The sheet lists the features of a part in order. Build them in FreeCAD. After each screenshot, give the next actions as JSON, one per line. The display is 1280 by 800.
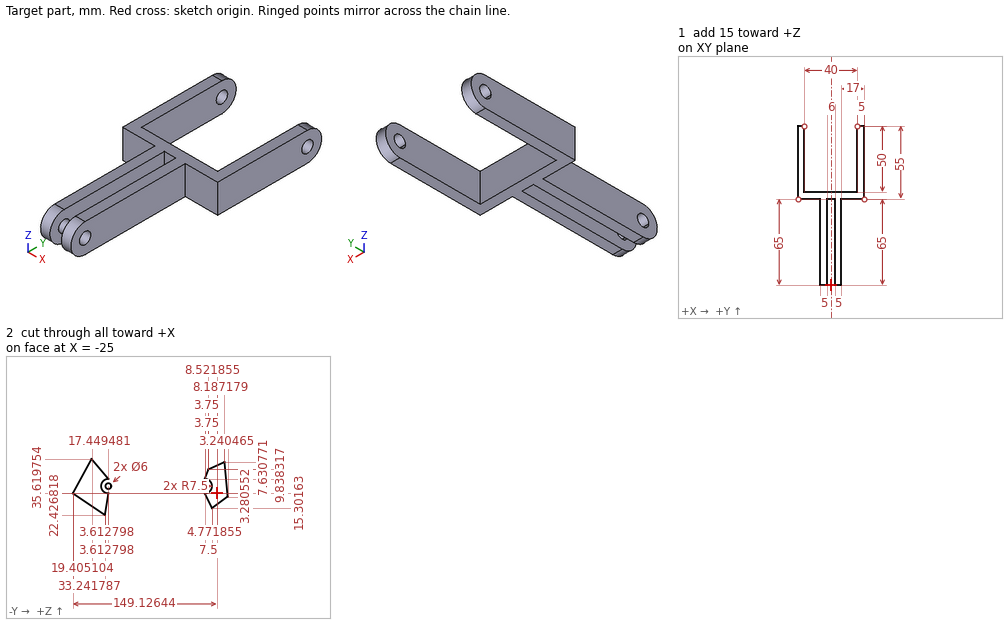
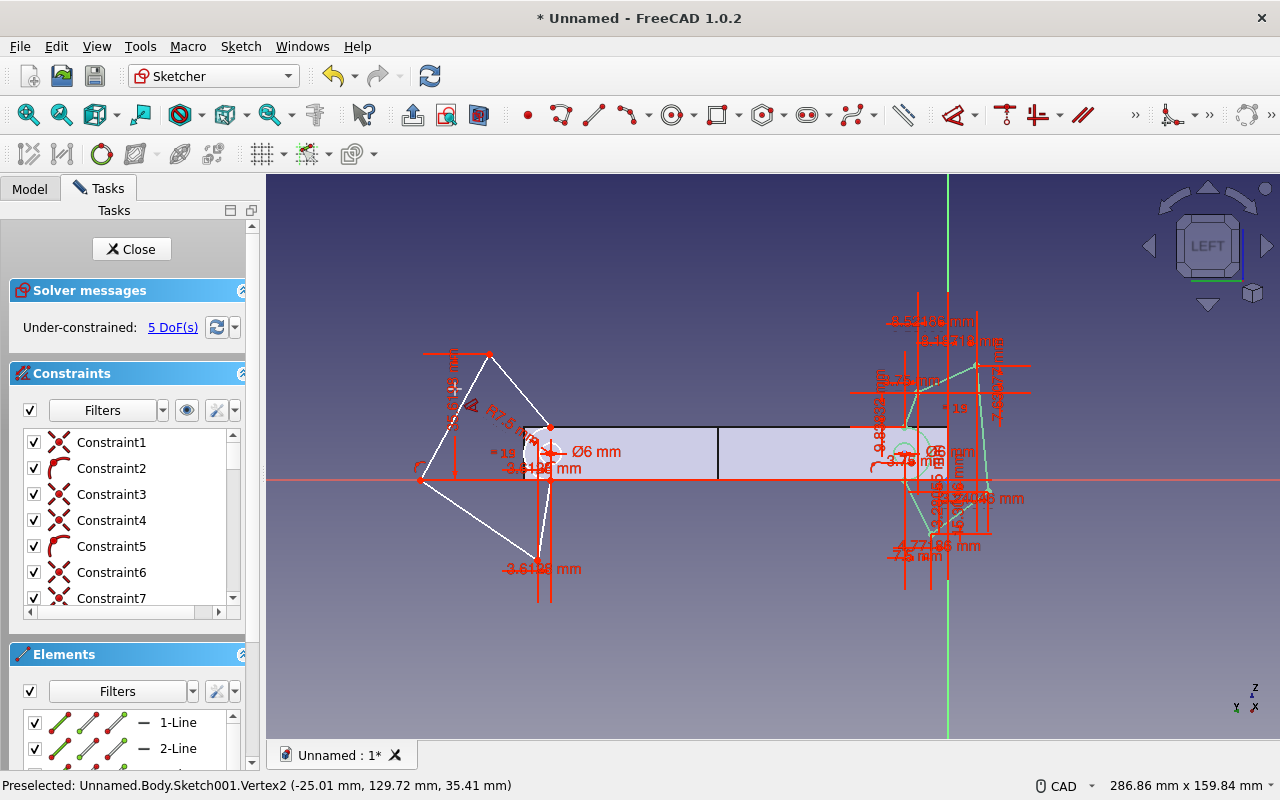
{"action": "left_click", "coordinate": [421, 480]}
{"action": "left_click", "coordinate": [684, 514]}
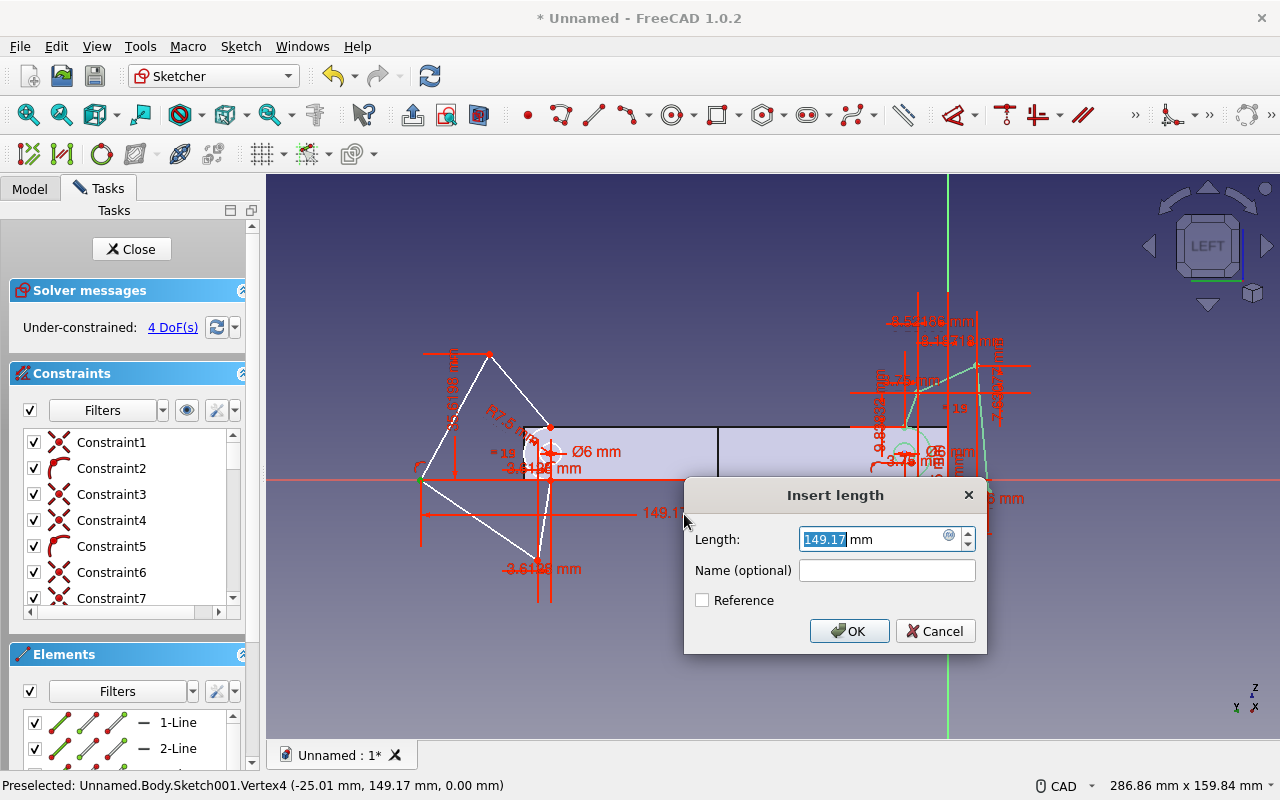
{"action": "type", "text": "149.12644"}
{"action": "key", "text": "Return"}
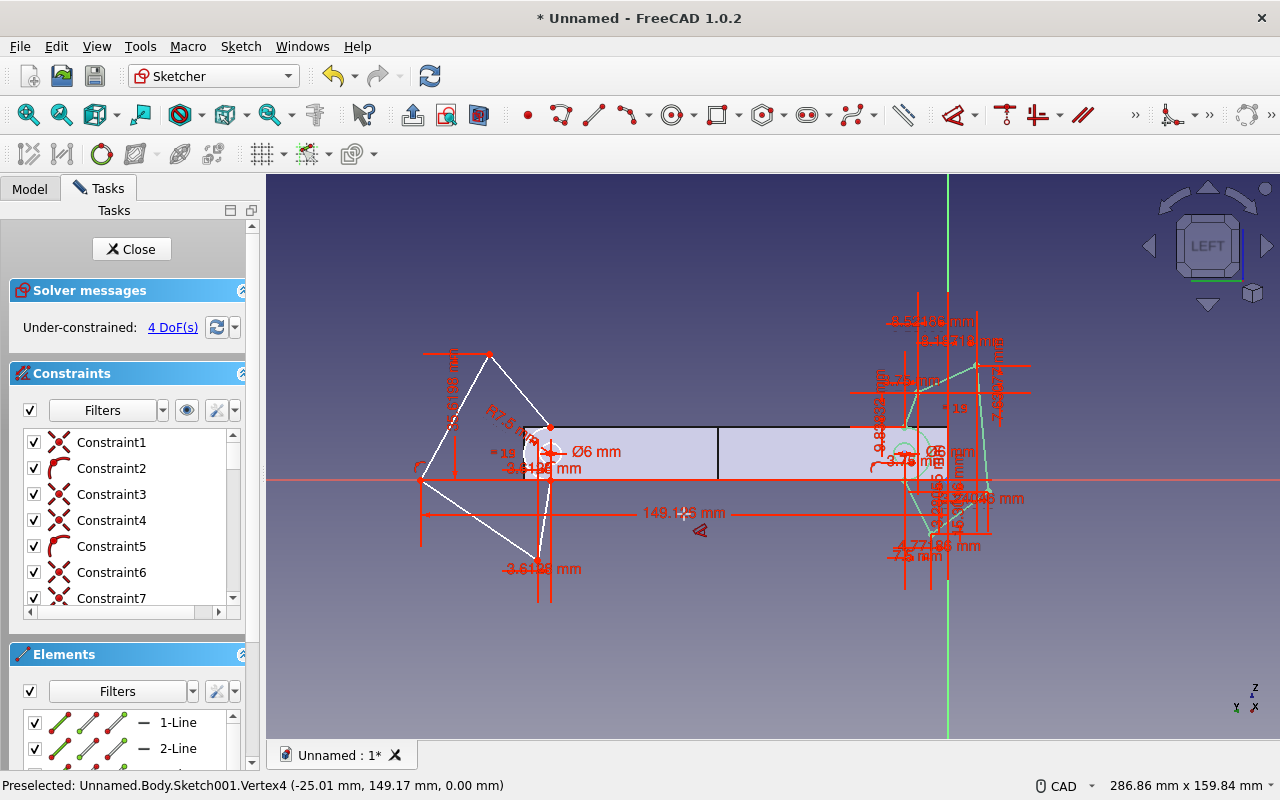
{"action": "left_click", "coordinate": [538, 561]}
{"action": "left_click", "coordinate": [982, 520]}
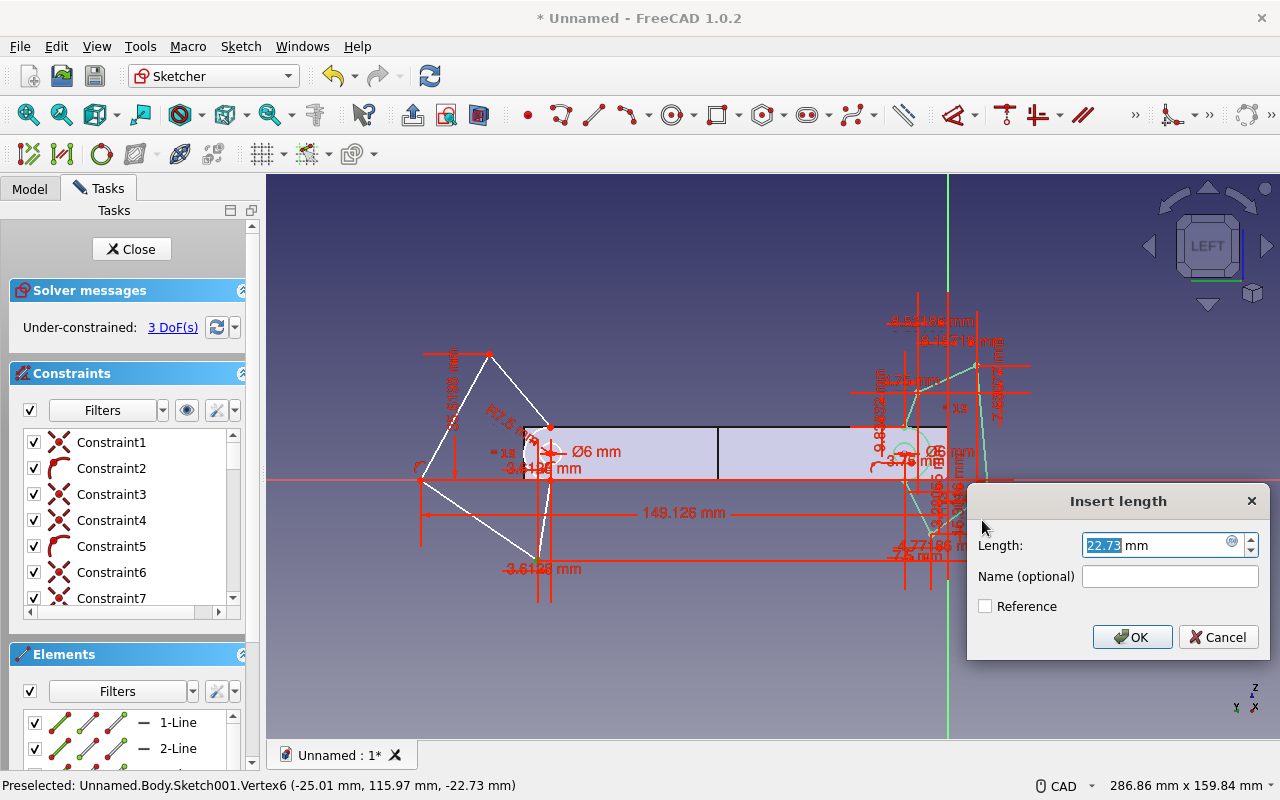
{"action": "type", "text": "22.426818"}
{"action": "key", "text": "Return"}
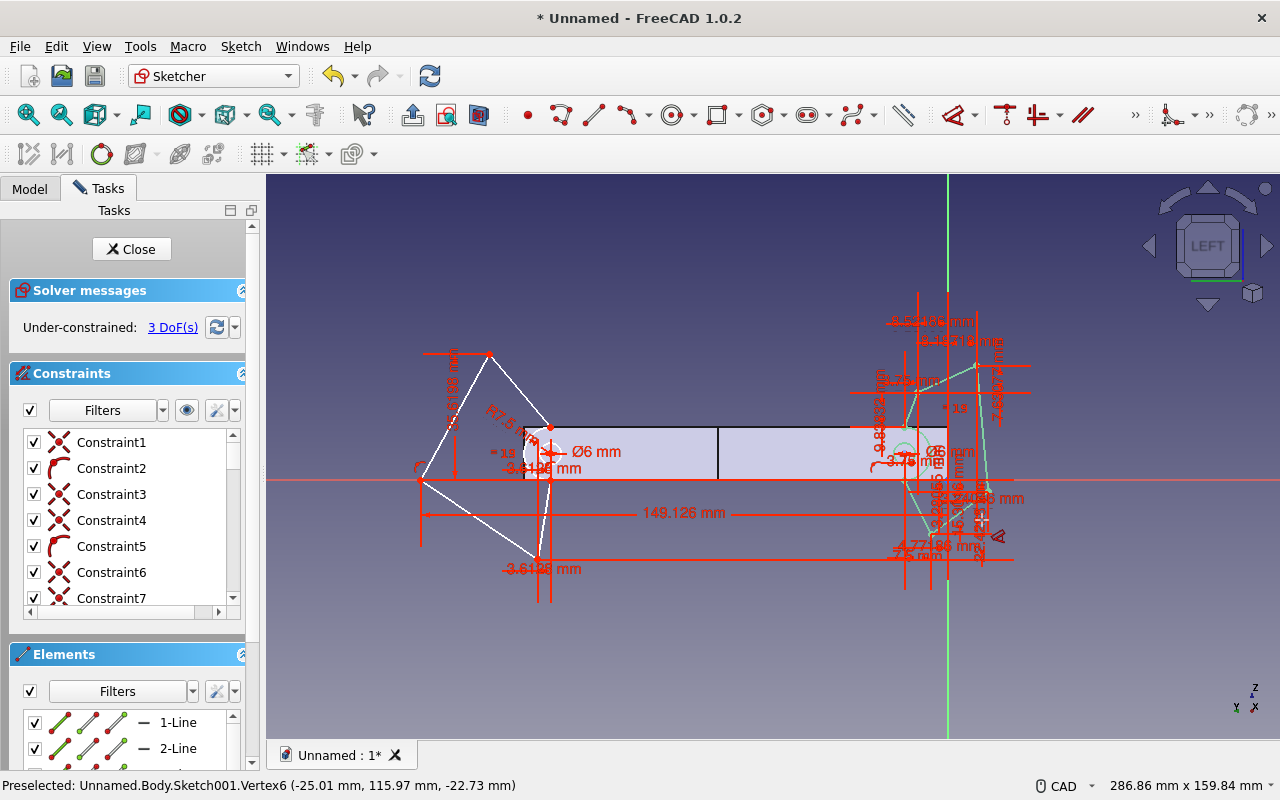
{"action": "left_click", "coordinate": [532, 405]}
{"action": "left_click", "coordinate": [520, 320]}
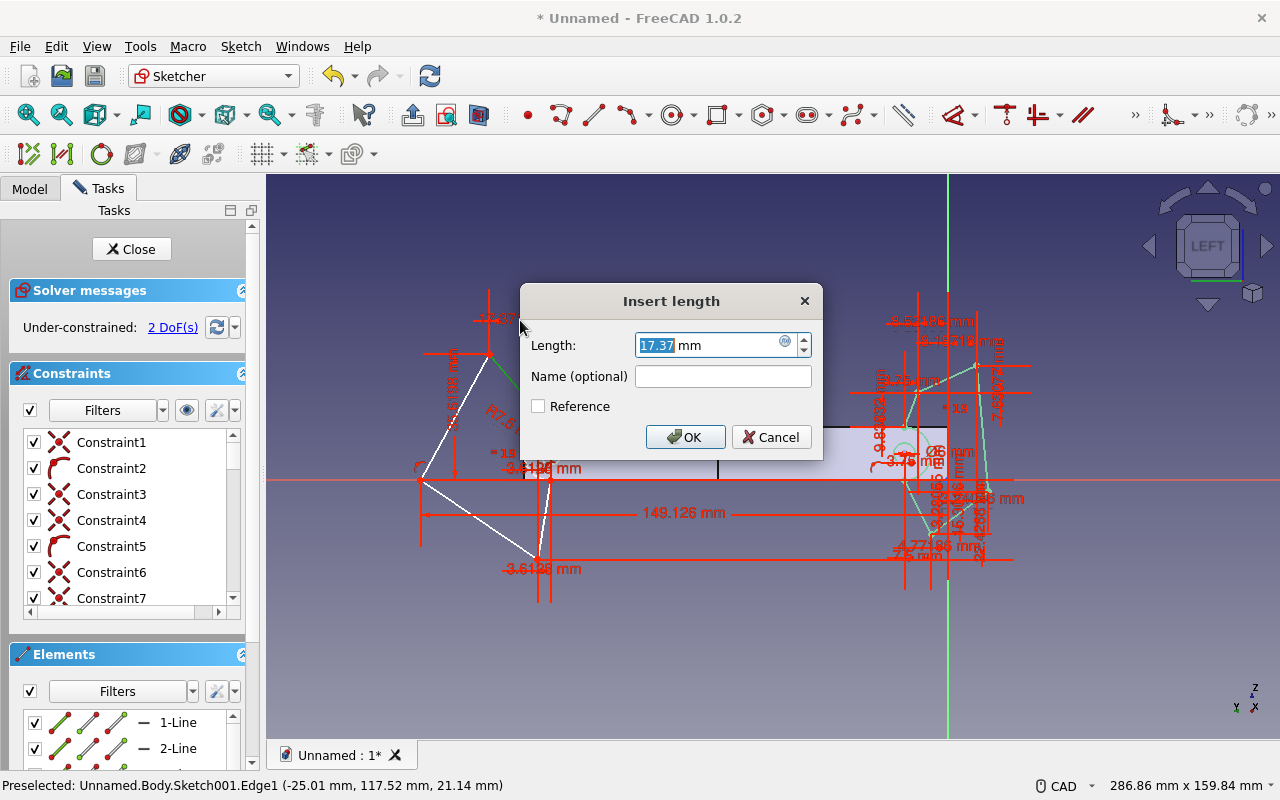
{"action": "type", "text": "17.449481"}
{"action": "key", "text": "Return"}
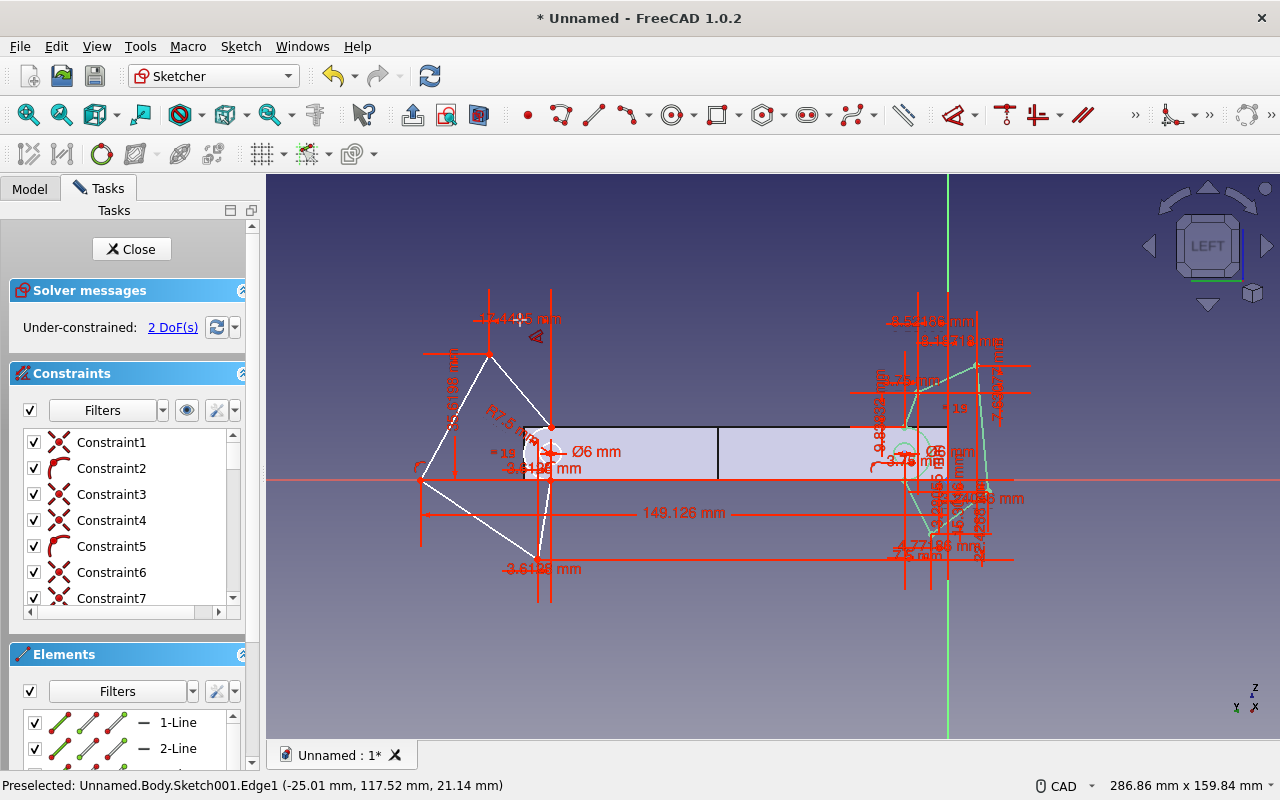
{"action": "left_click", "coordinate": [469, 392]}
{"action": "left_click", "coordinate": [439, 320]}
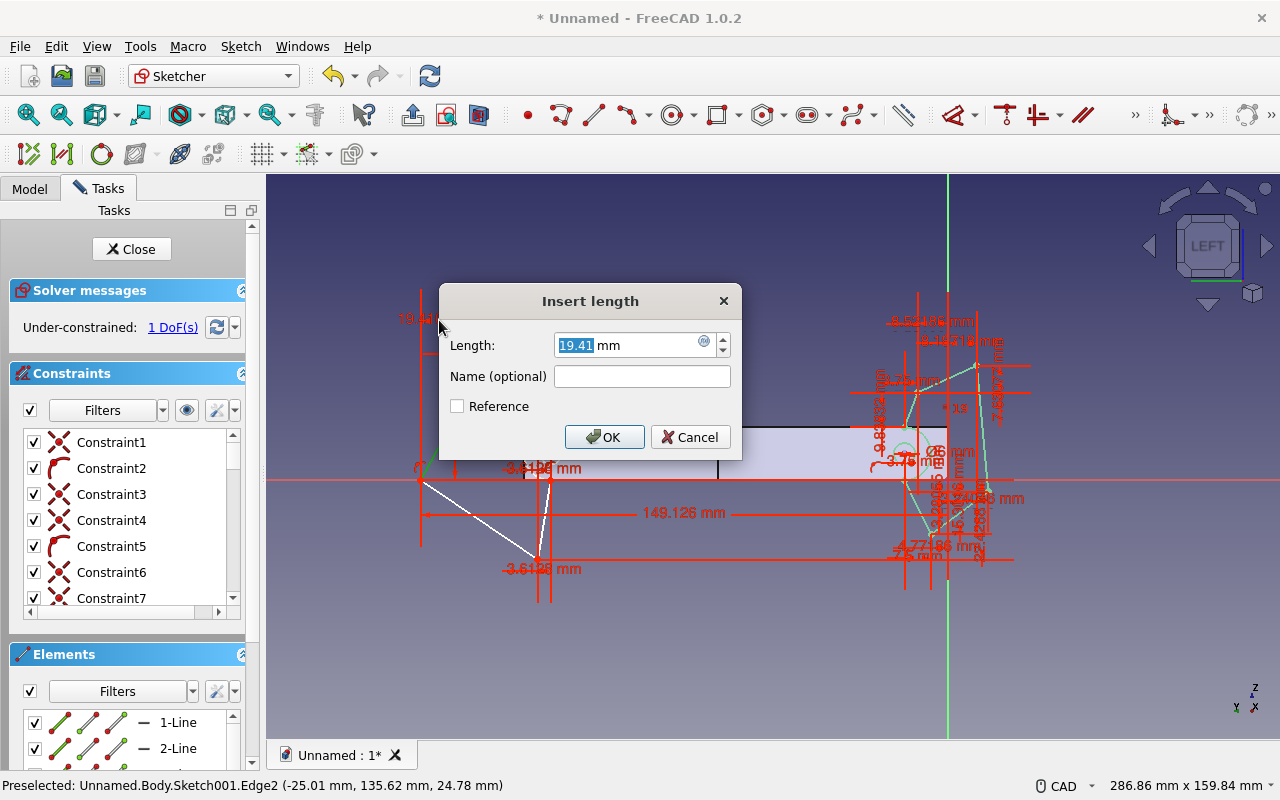
{"action": "type", "text": "19.405104"}
{"action": "key", "text": "Return"}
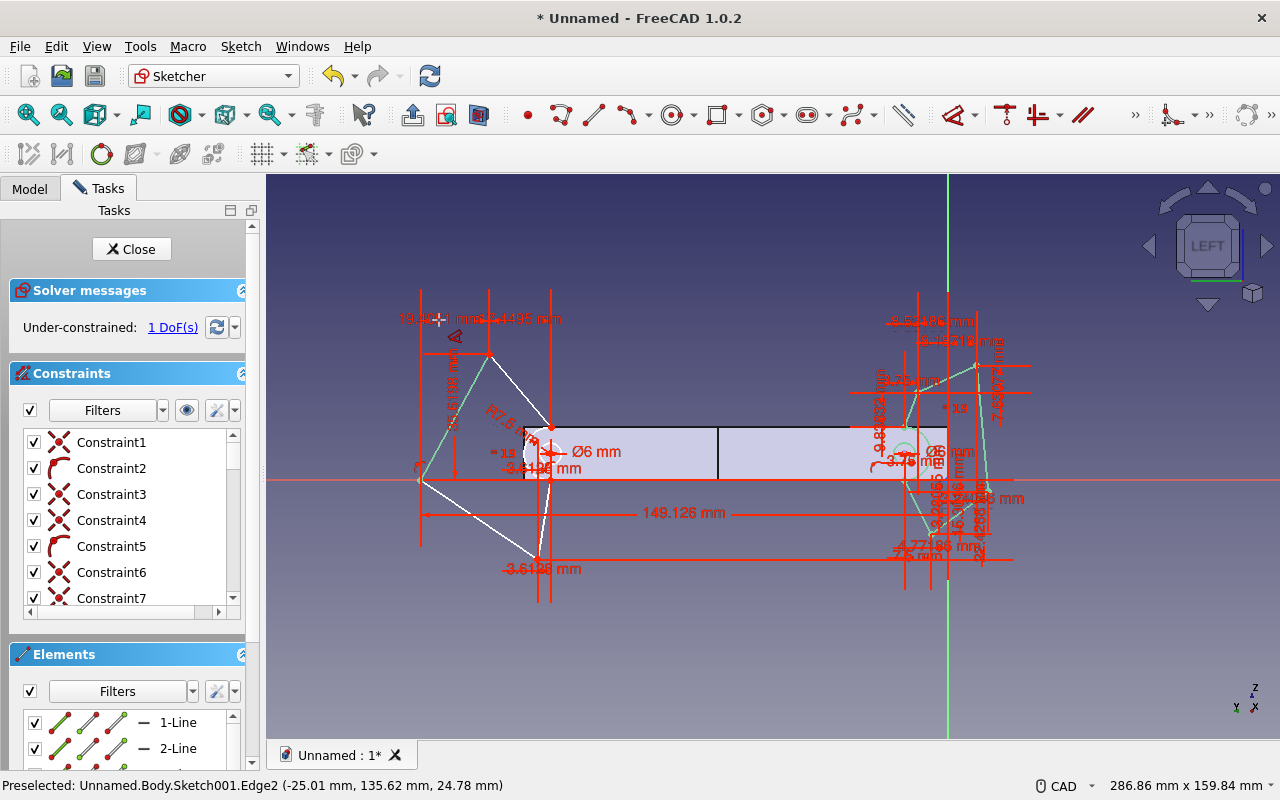
{"action": "left_click", "coordinate": [456, 504]}
{"action": "left_click", "coordinate": [479, 594]}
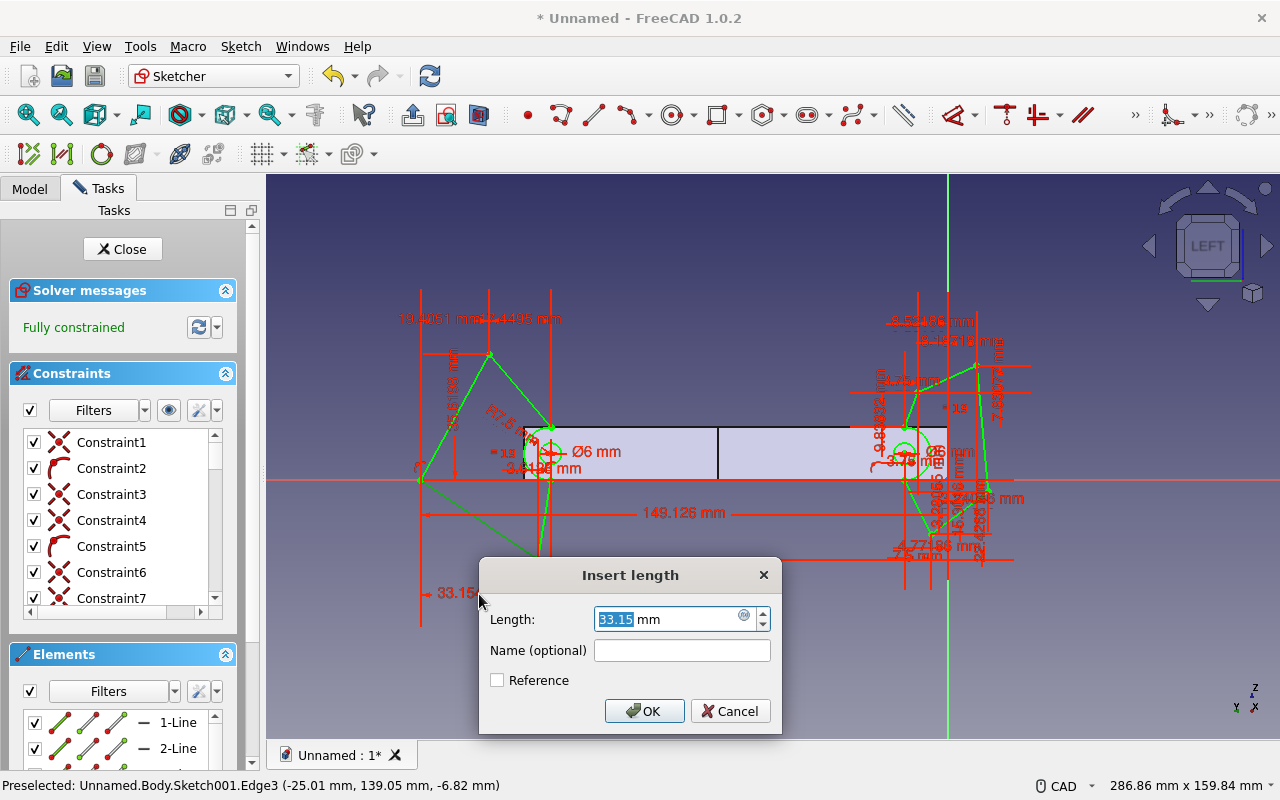
{"action": "type", "text": "33.241787"}
{"action": "key", "text": "Return"}
{"action": "key", "text": "Escape"}